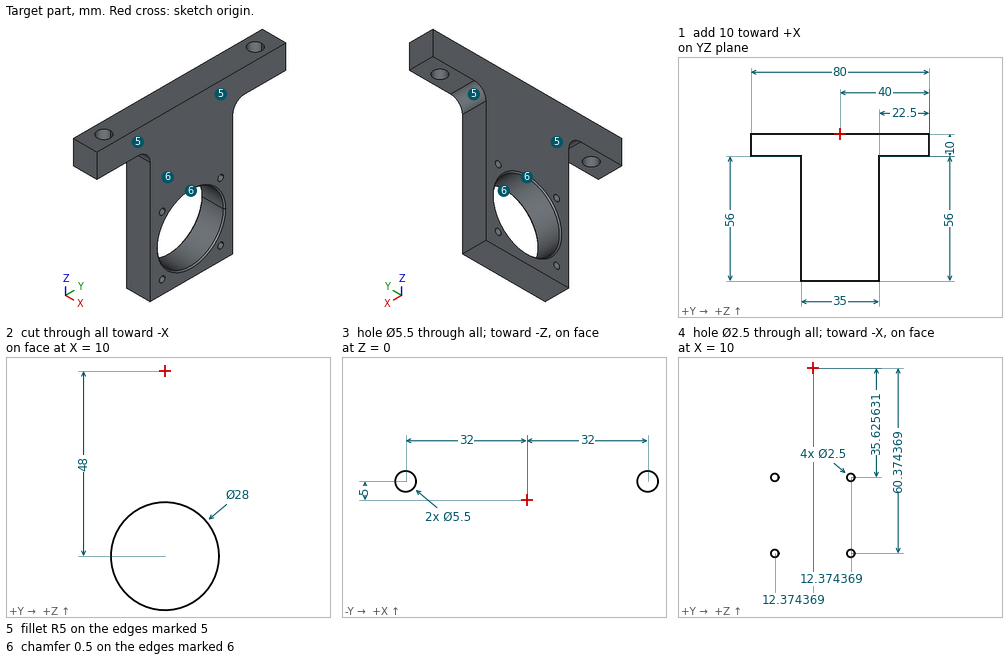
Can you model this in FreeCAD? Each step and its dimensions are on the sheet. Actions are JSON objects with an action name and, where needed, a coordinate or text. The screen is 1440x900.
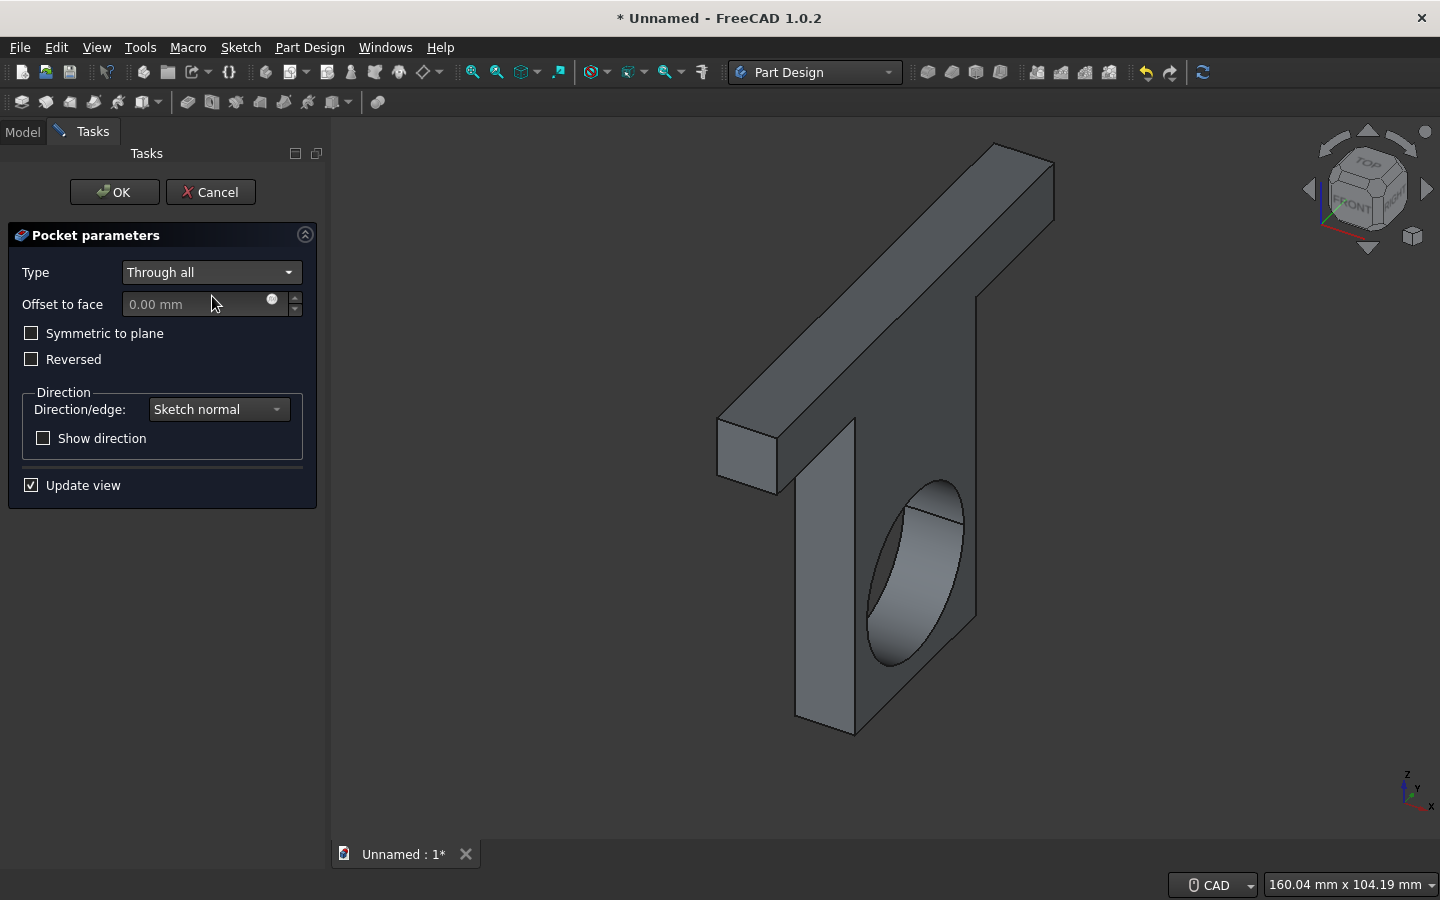
{"action": "left_click", "coordinate": [115, 192]}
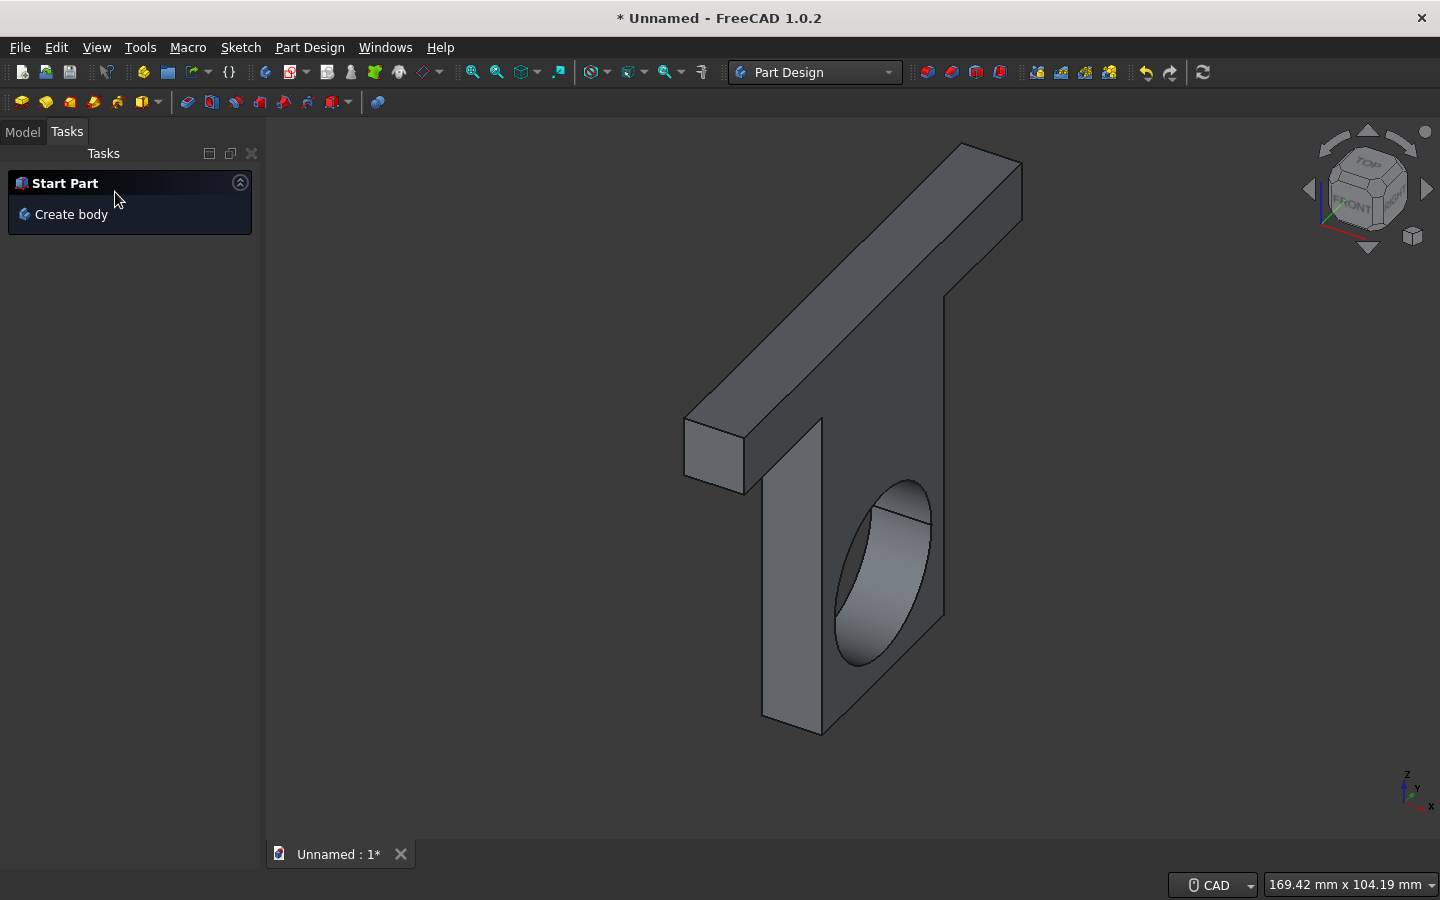
{"action": "left_click", "coordinate": [972, 172]}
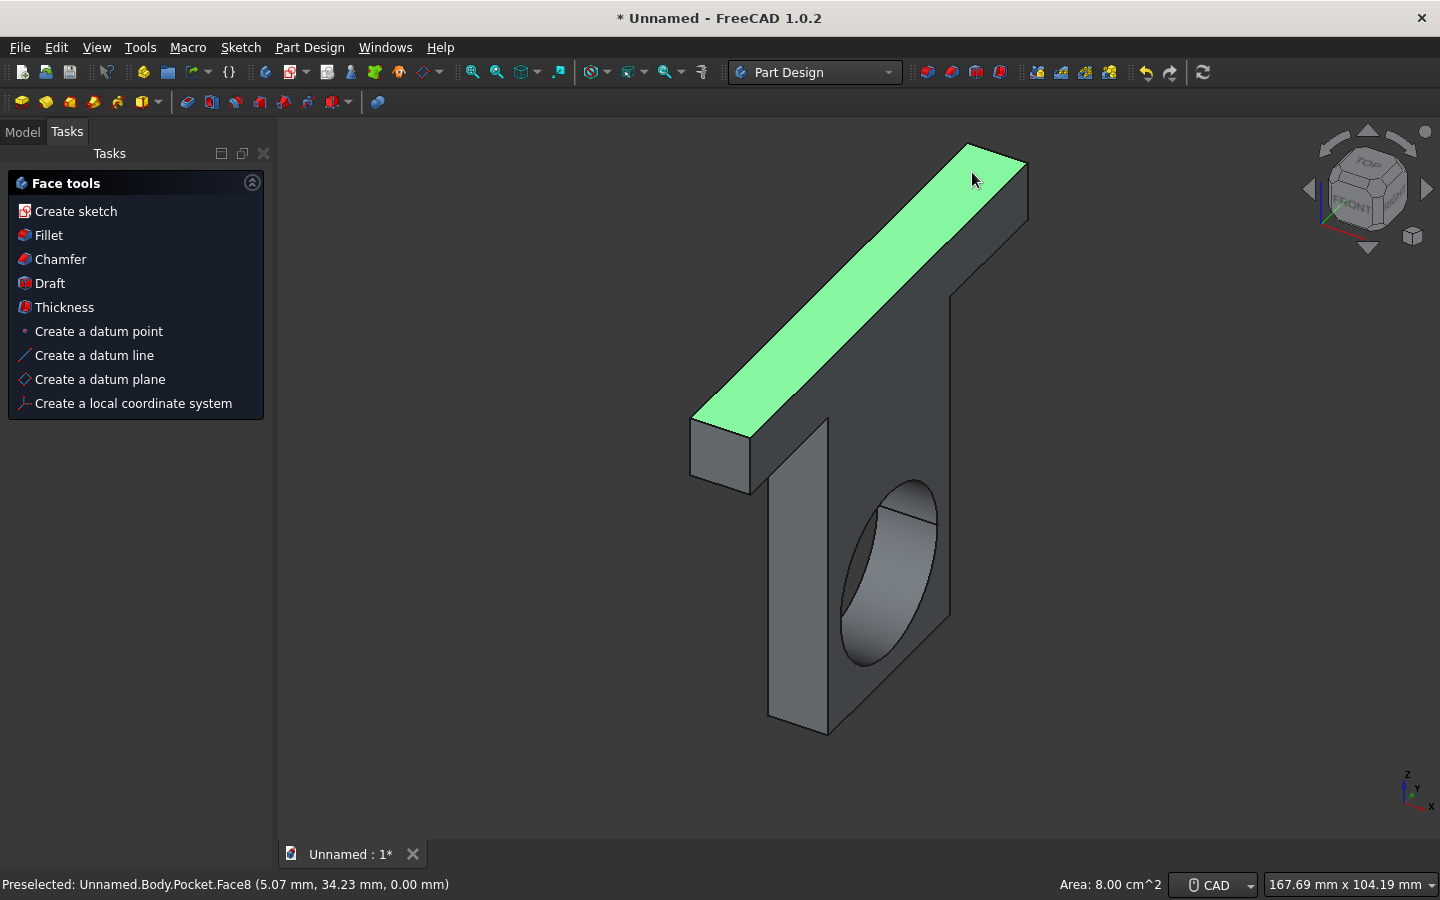
{"action": "left_click", "coordinate": [290, 72]}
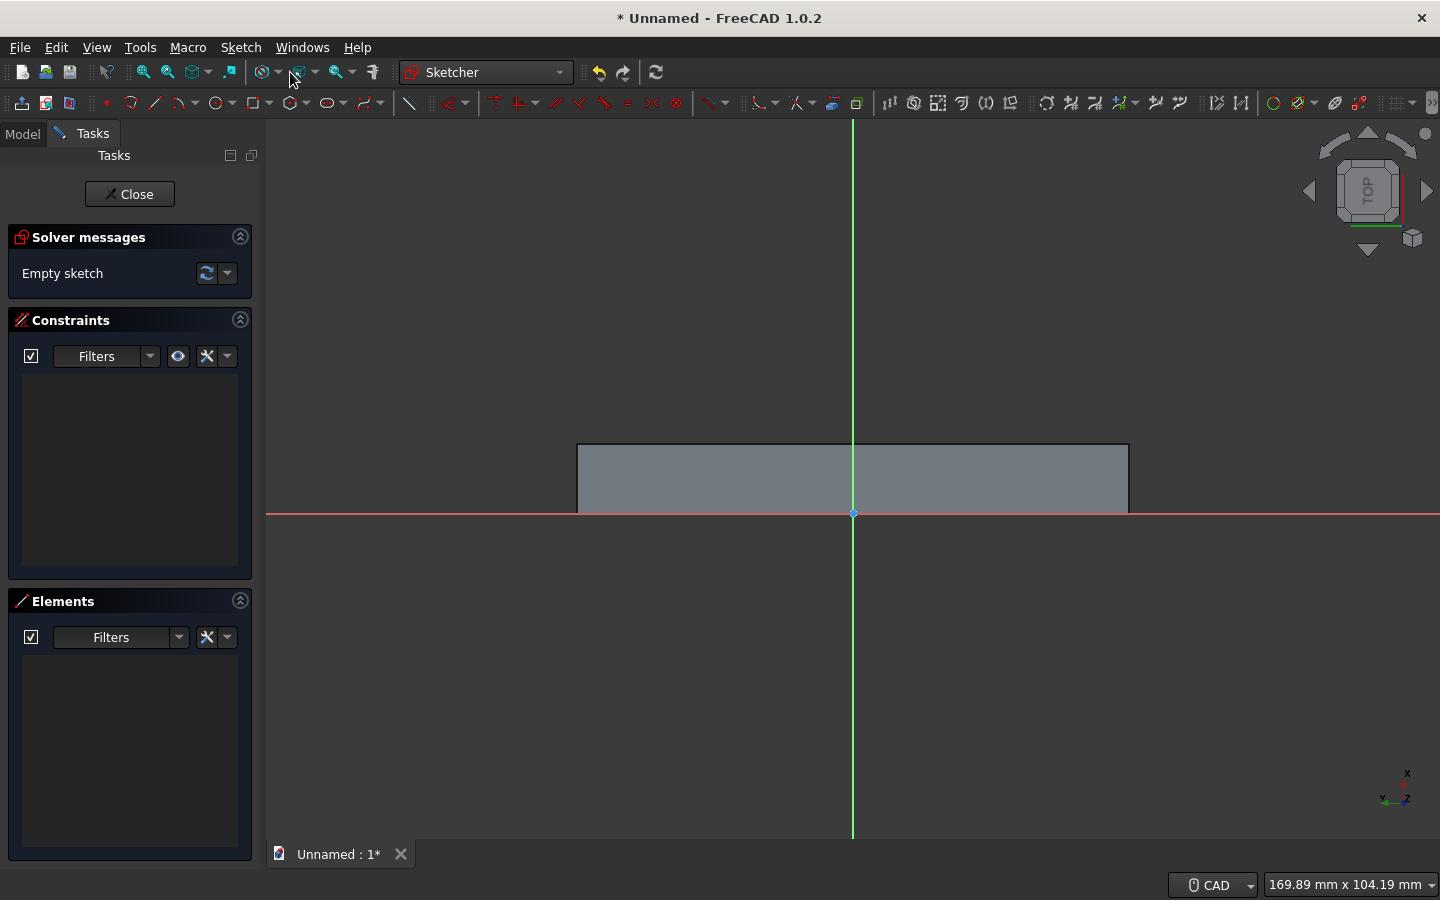
{"action": "scroll", "coordinate": [992, 503], "scroll_direction": "up", "scroll_amount": 2}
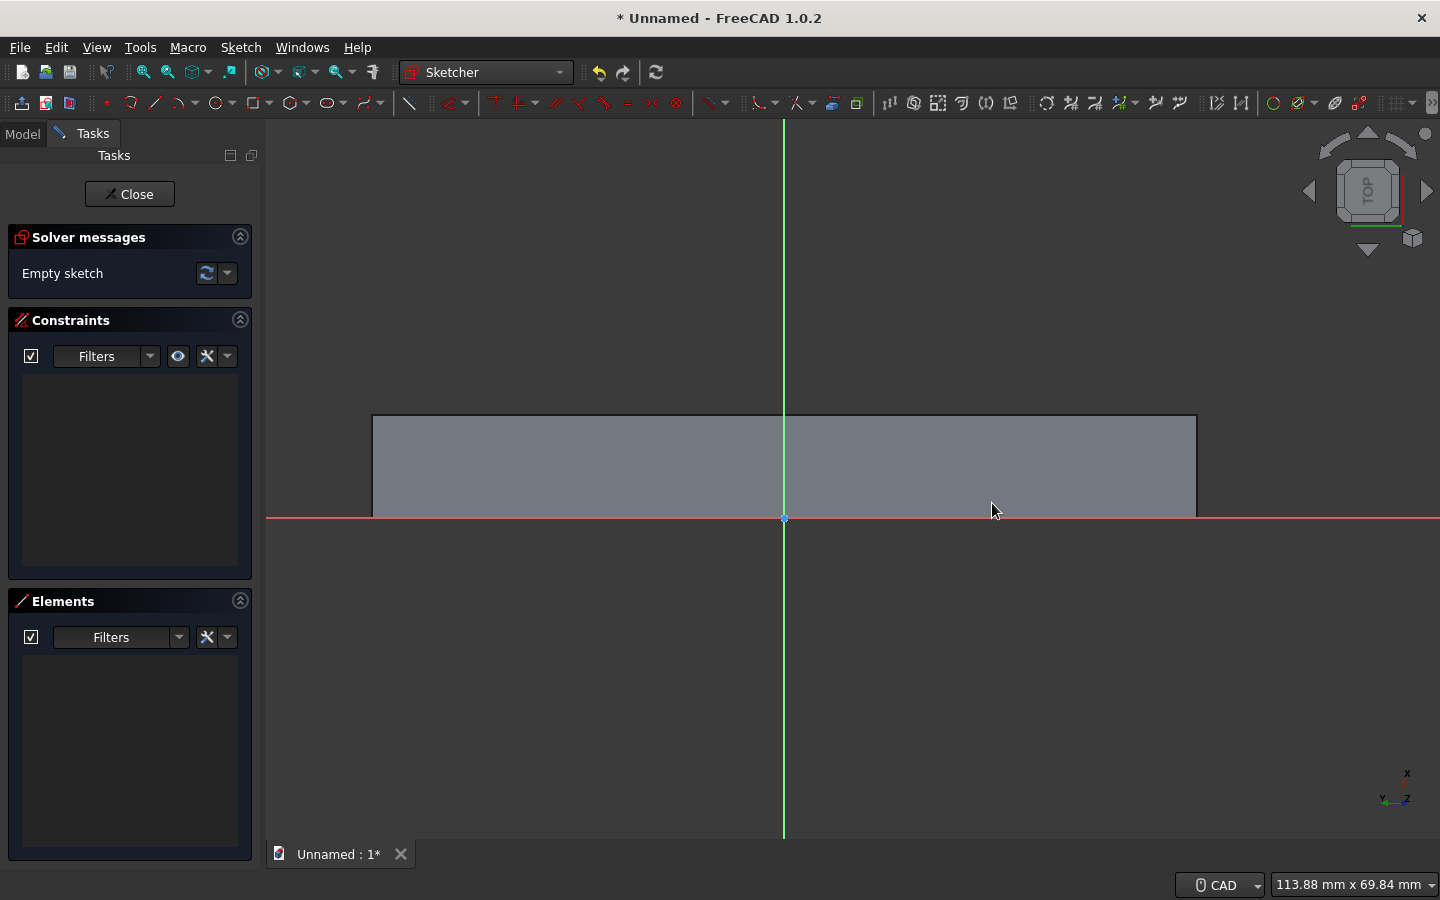
{"action": "left_click", "coordinate": [216, 104]}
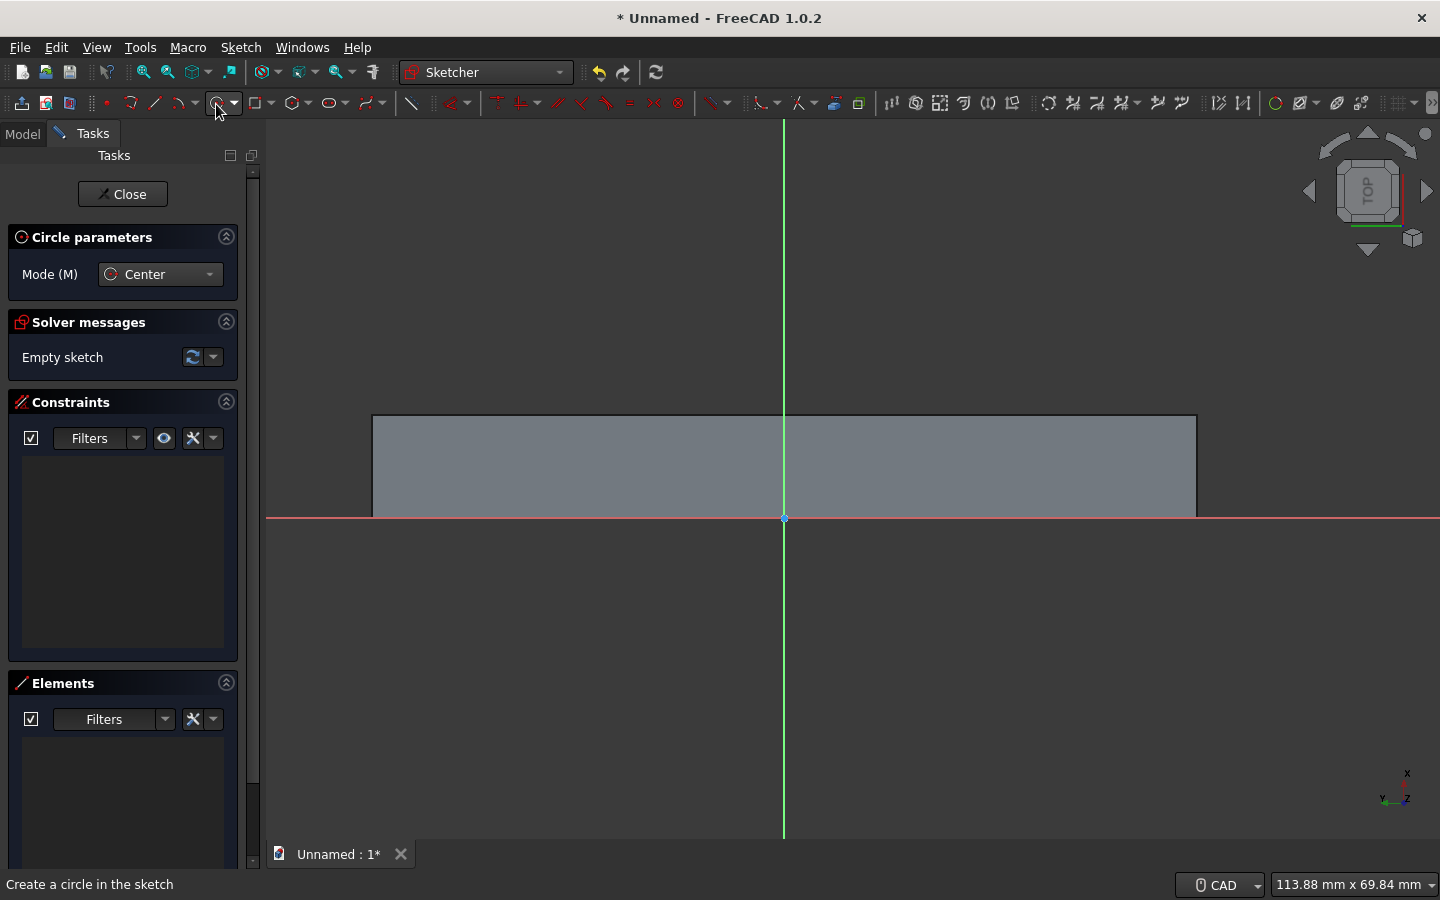
{"action": "left_click", "coordinate": [454, 467]}
{"action": "mouse_move", "coordinate": [474, 447]}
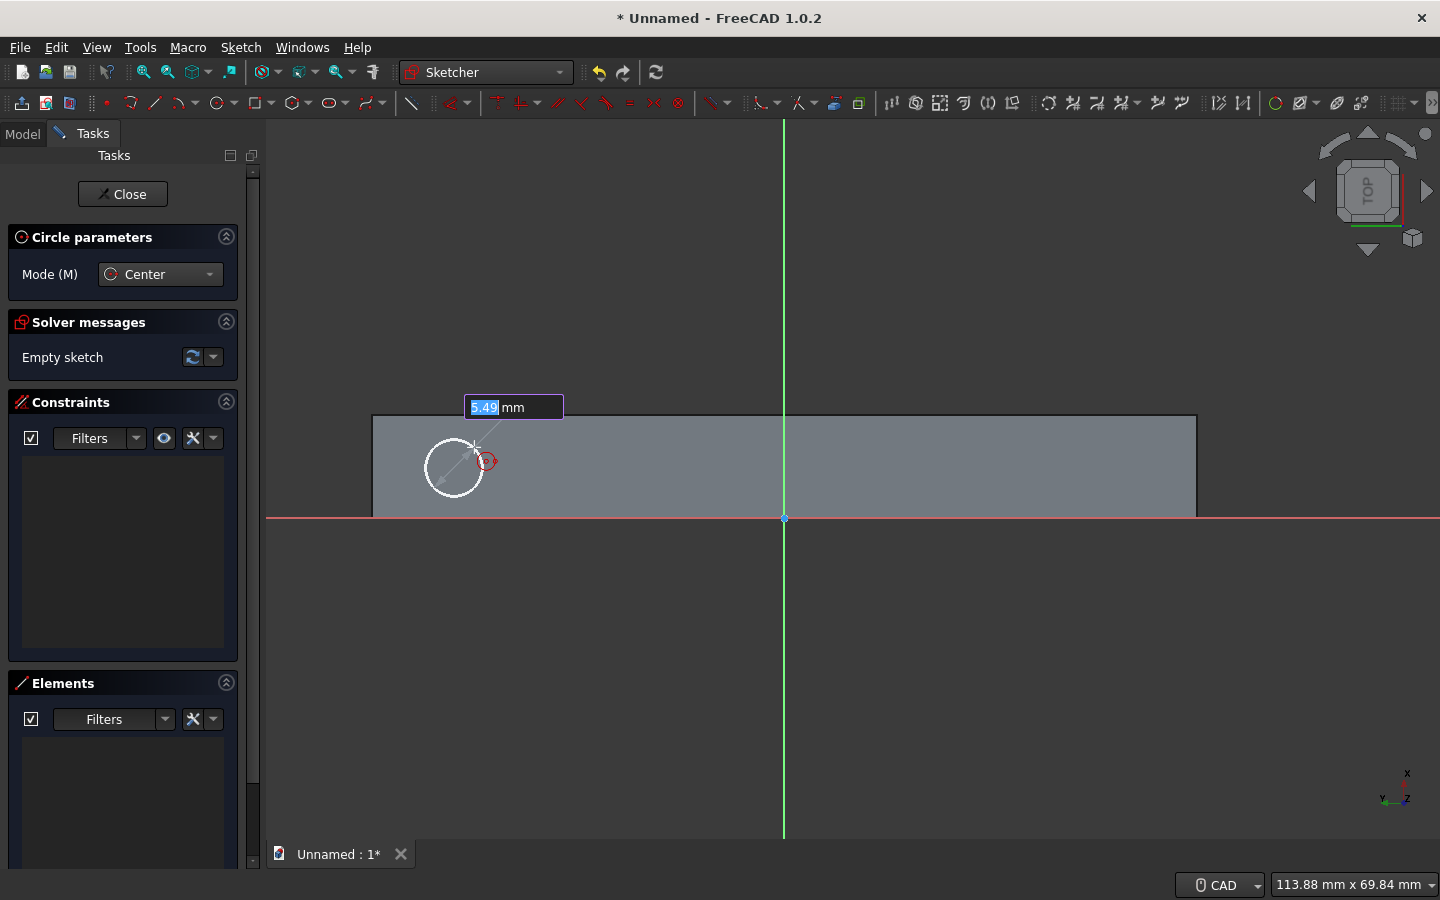
{"action": "type", "text": "5.5"}
{"action": "key", "text": "Return"}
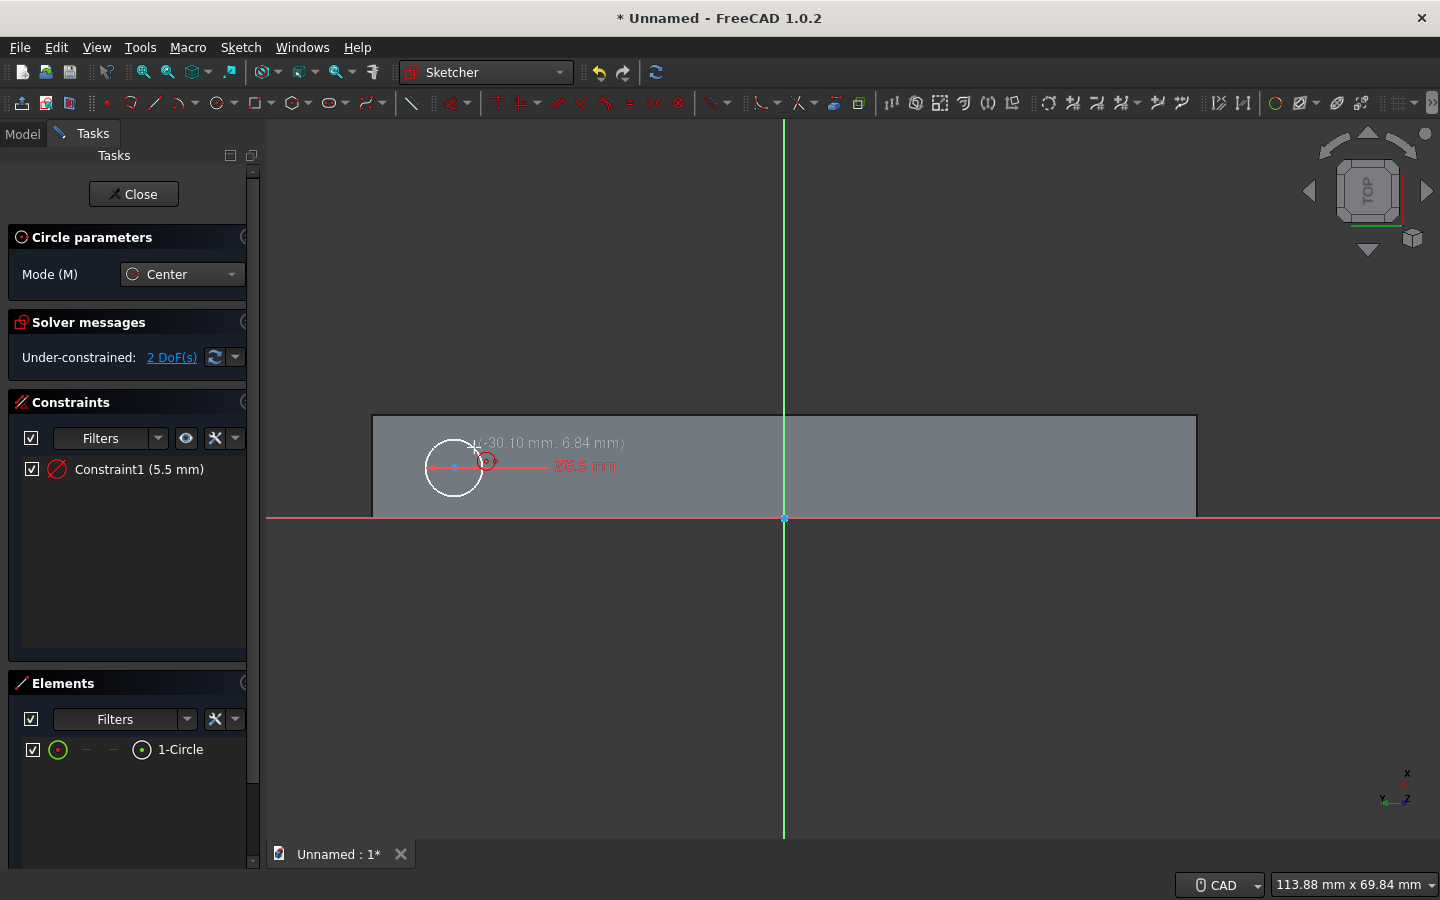
{"action": "left_click", "coordinate": [1114, 467]}
{"action": "mouse_move", "coordinate": [1134, 447]}